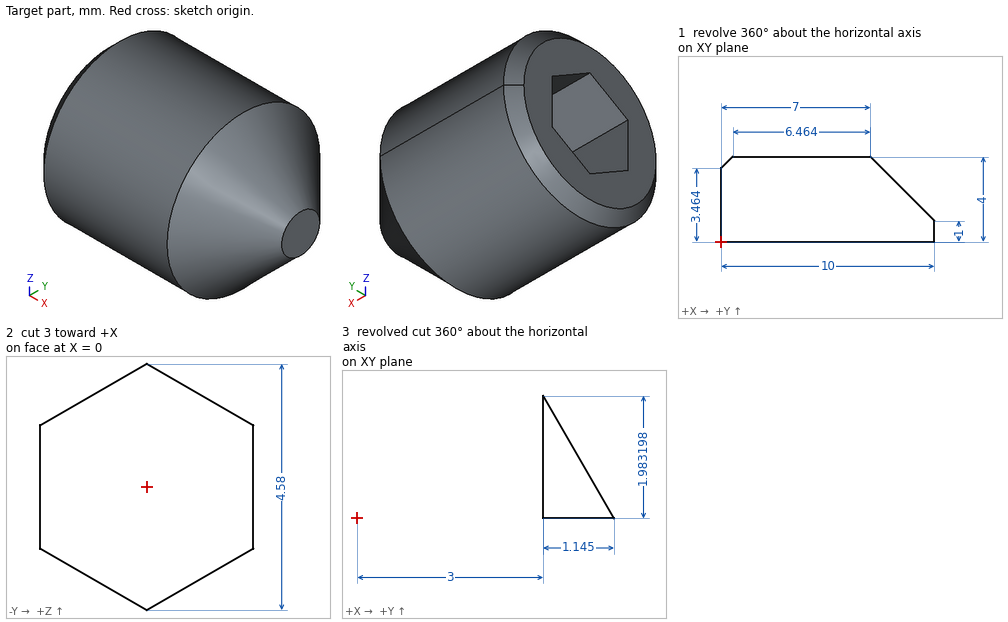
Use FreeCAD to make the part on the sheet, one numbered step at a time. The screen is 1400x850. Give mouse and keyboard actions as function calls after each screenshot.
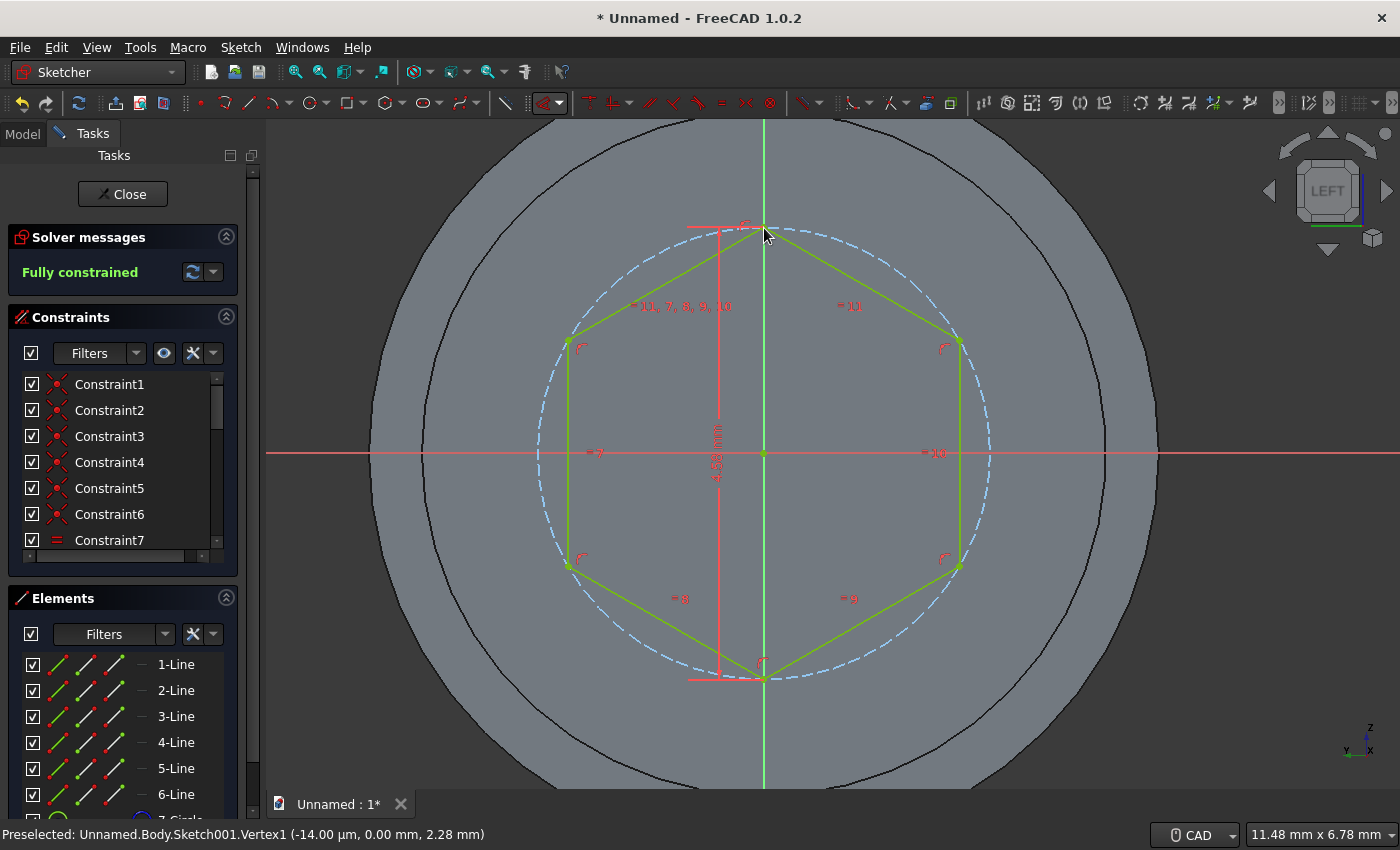
click(123, 194)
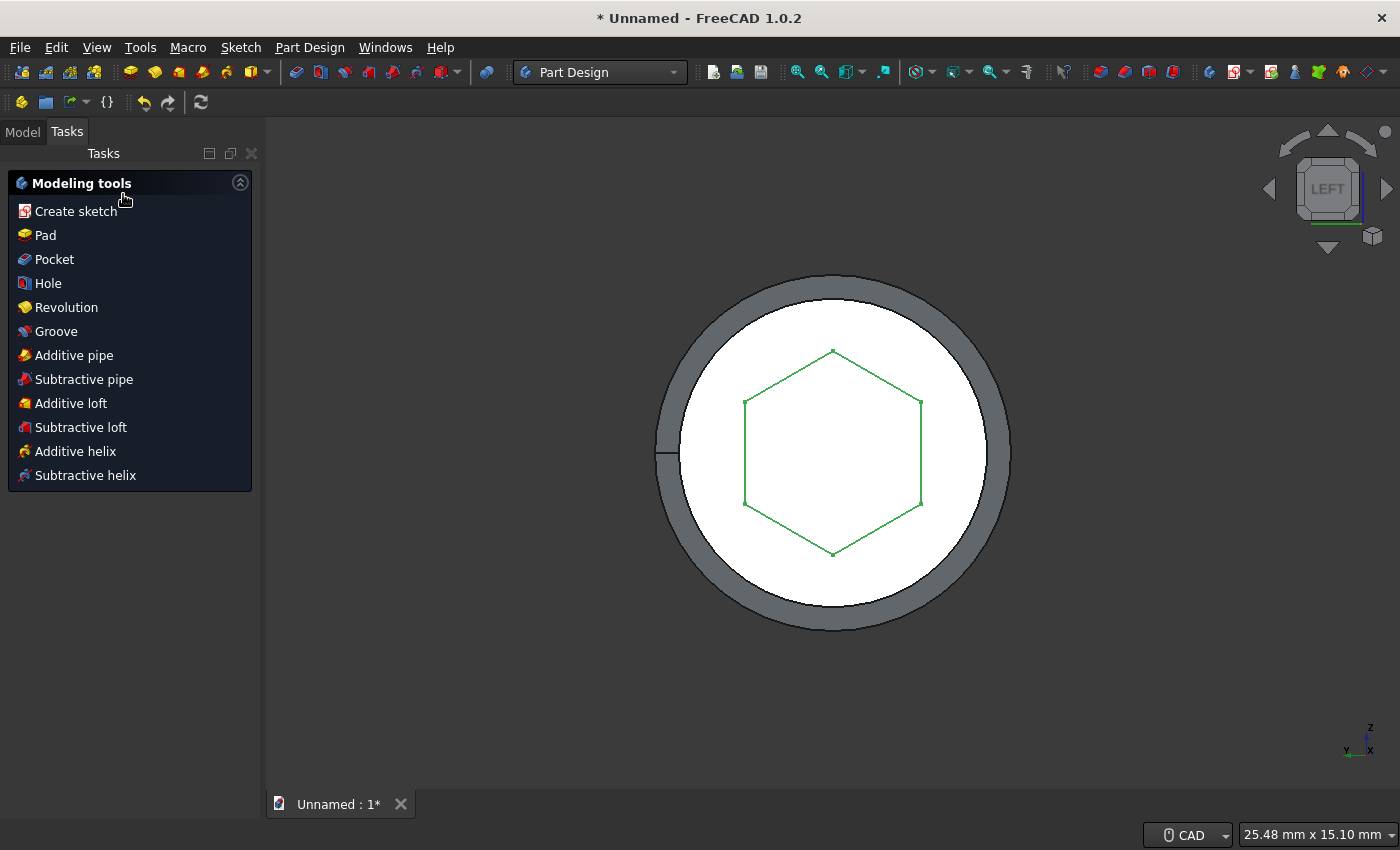
click(298, 72)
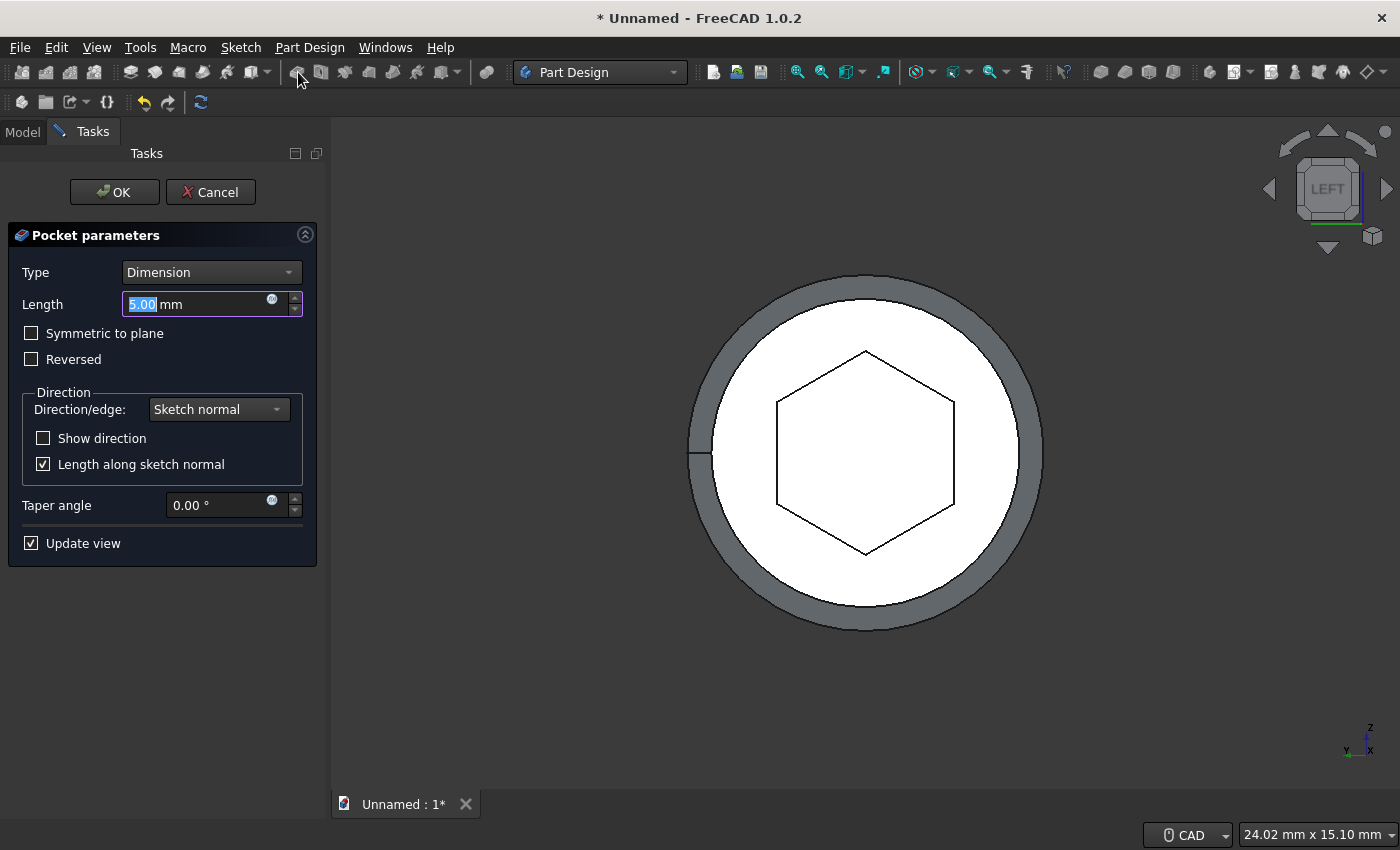
text(3)
key(Tab)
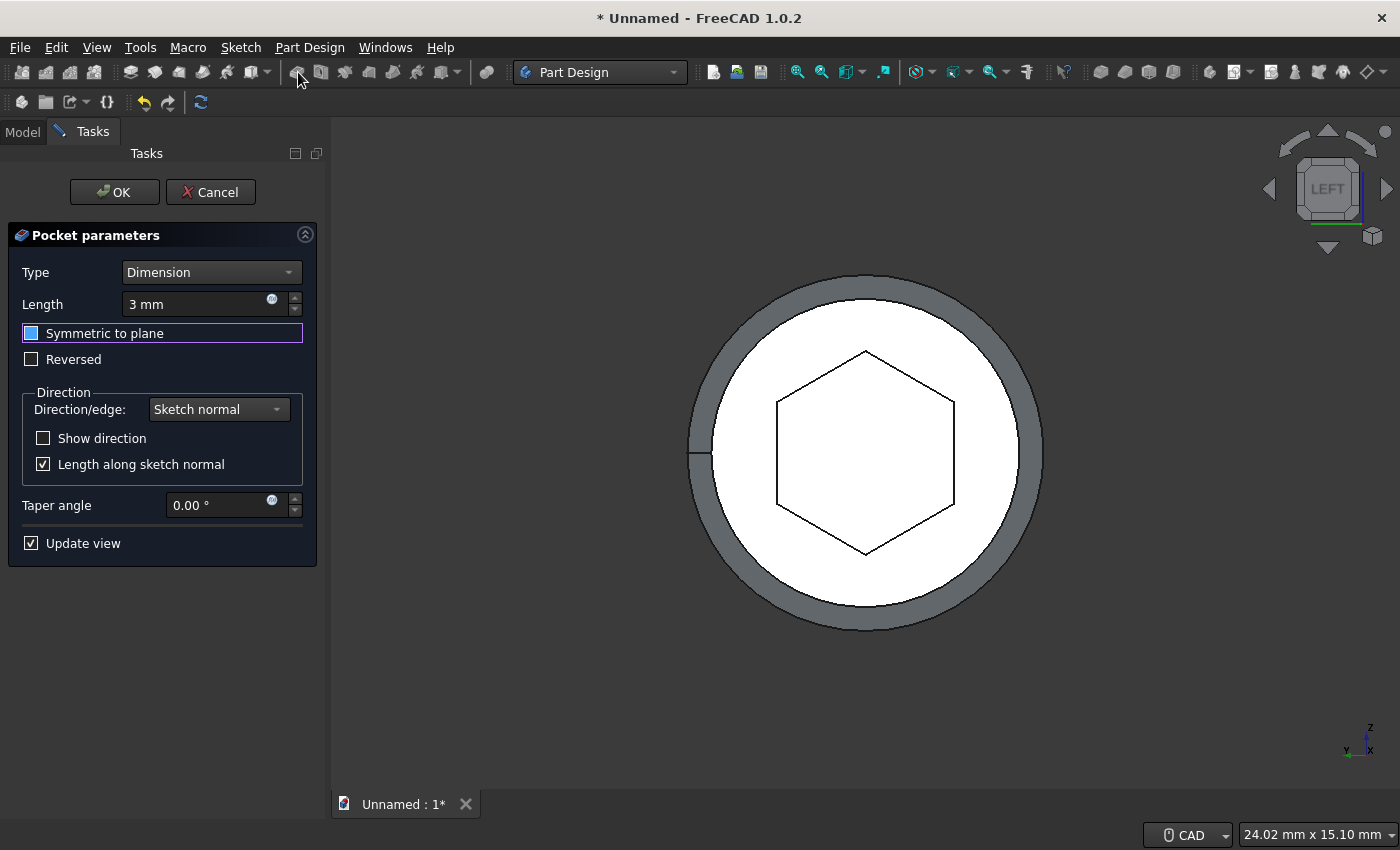
click(115, 192)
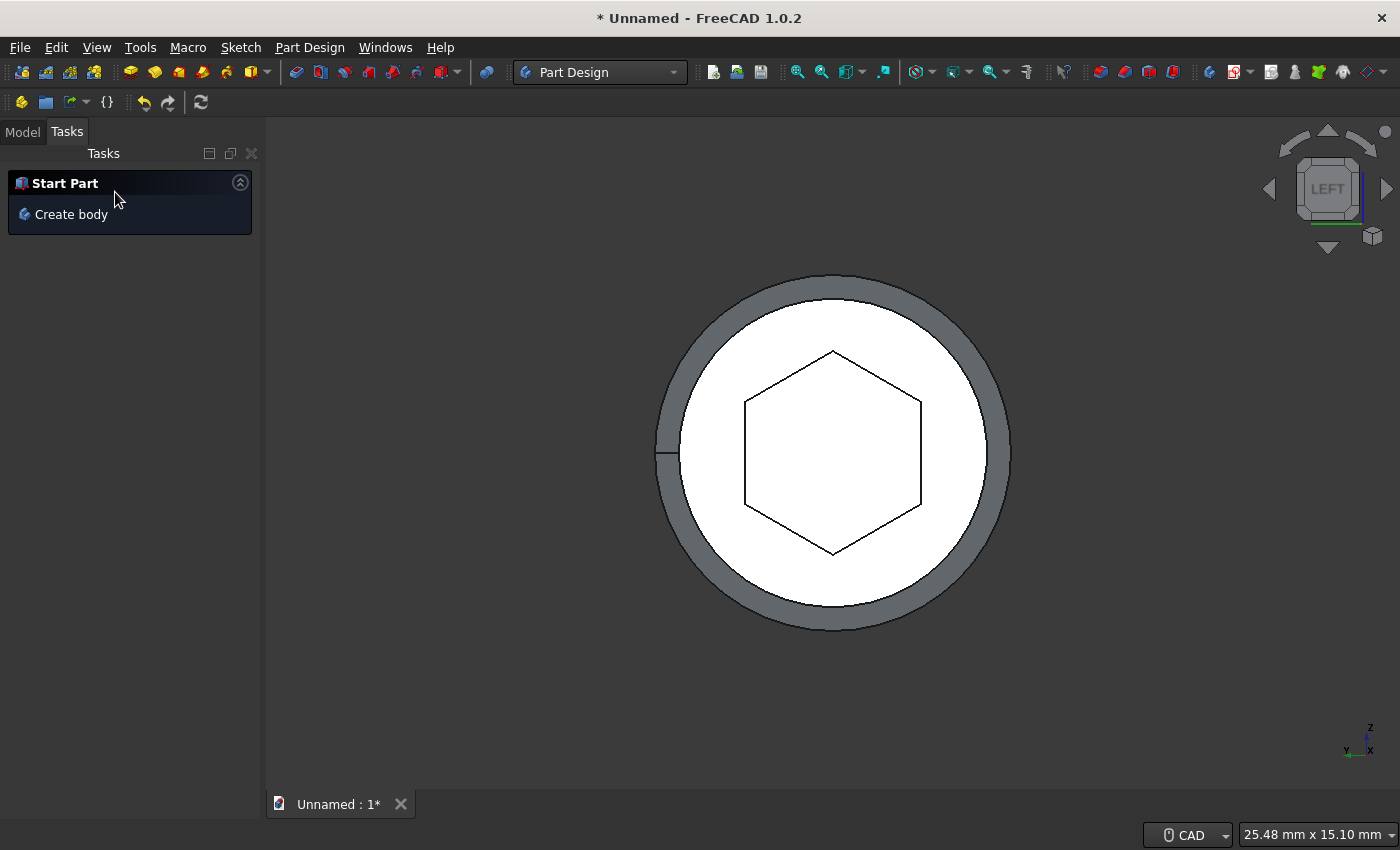
click(1234, 72)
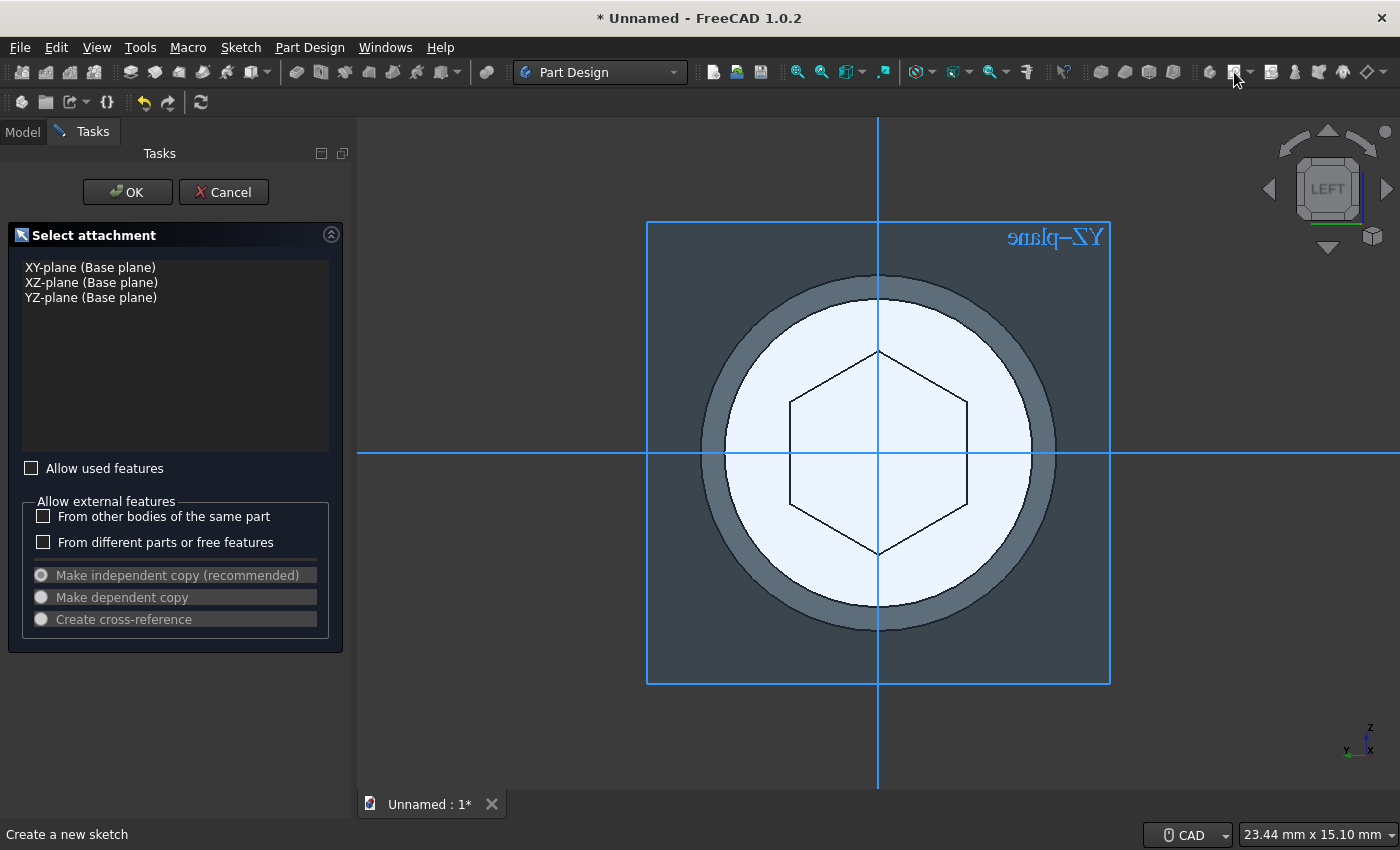
click(82, 268)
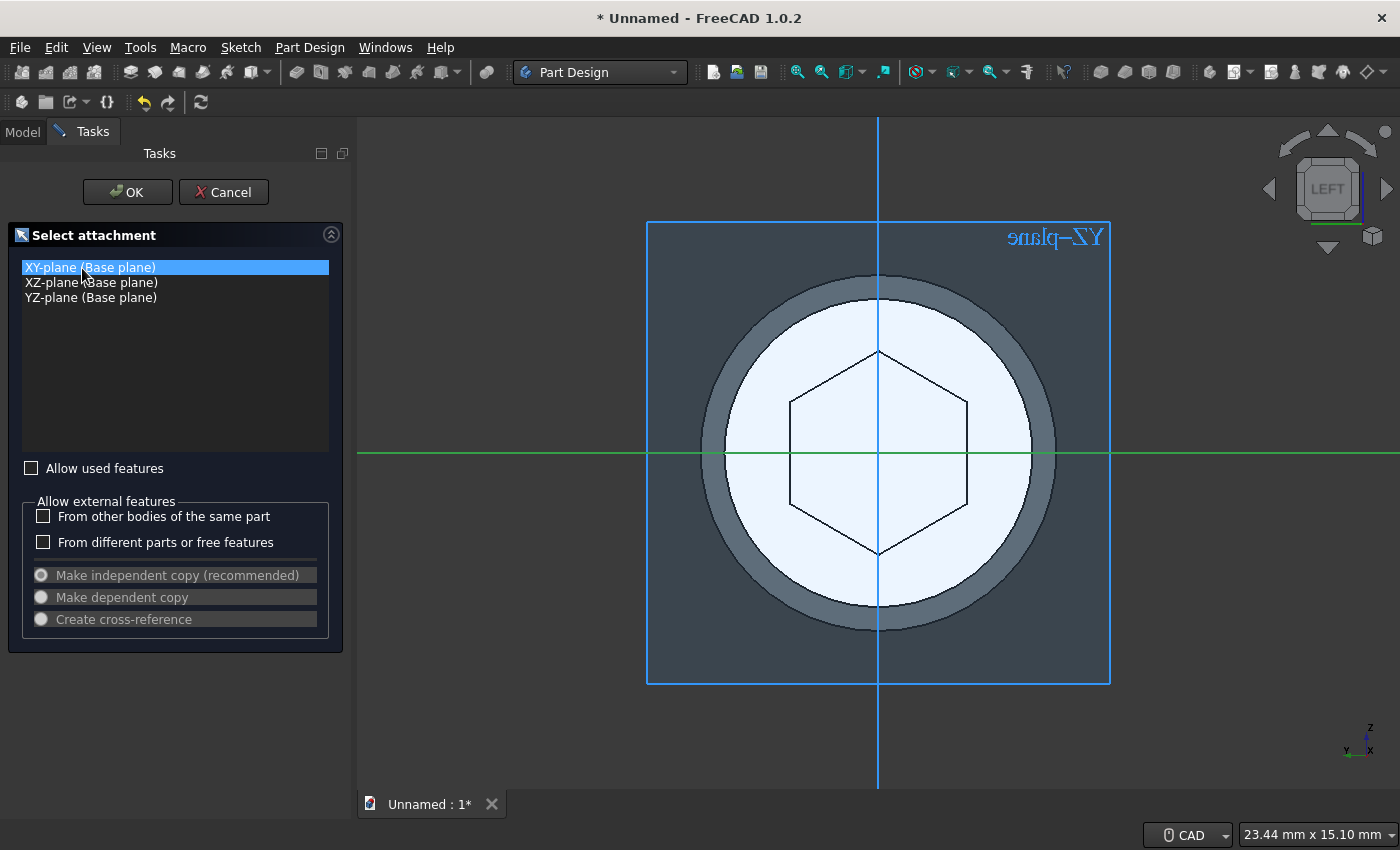
click(128, 192)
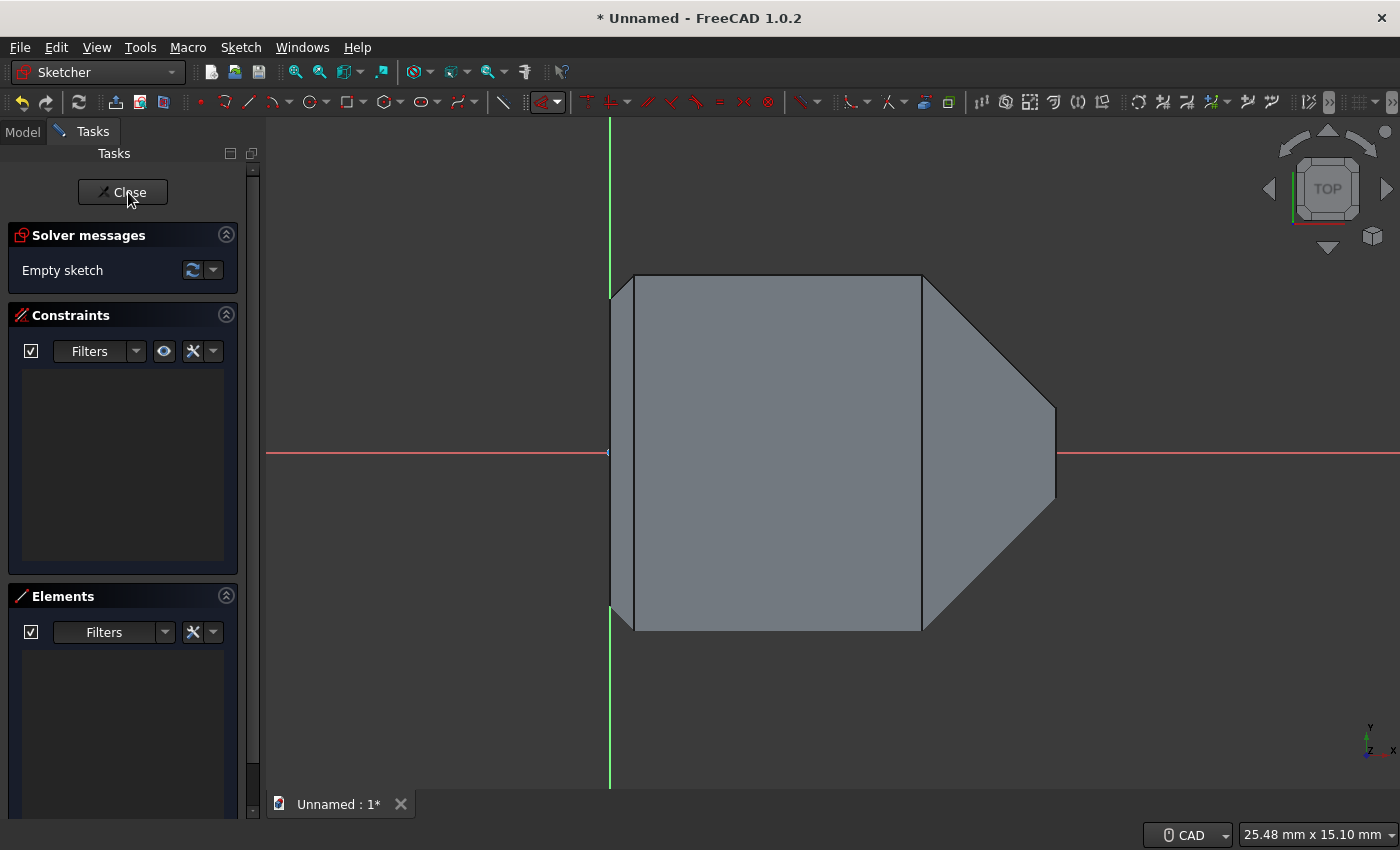
click(164, 102)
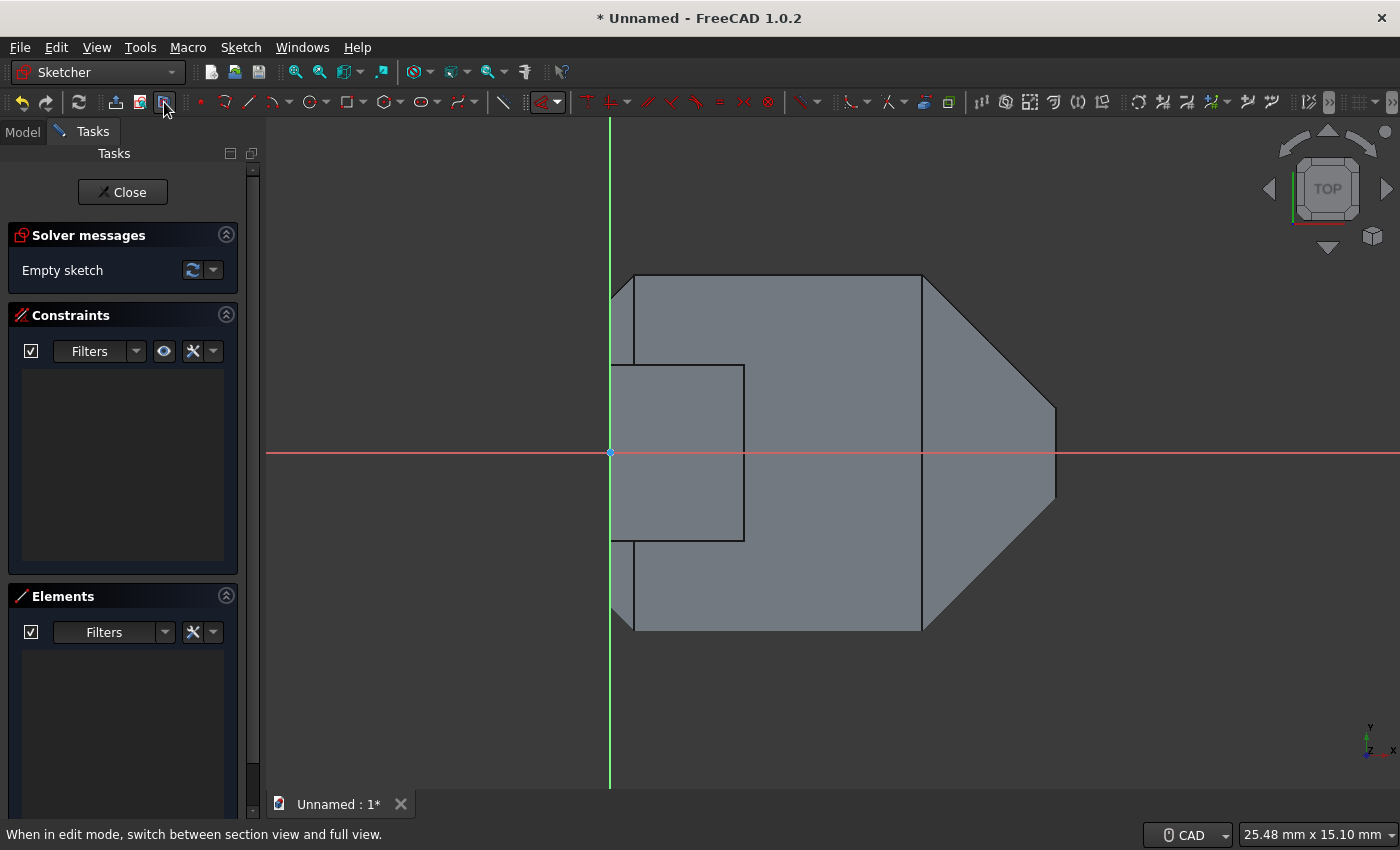
scroll(676, 390, up, 6)